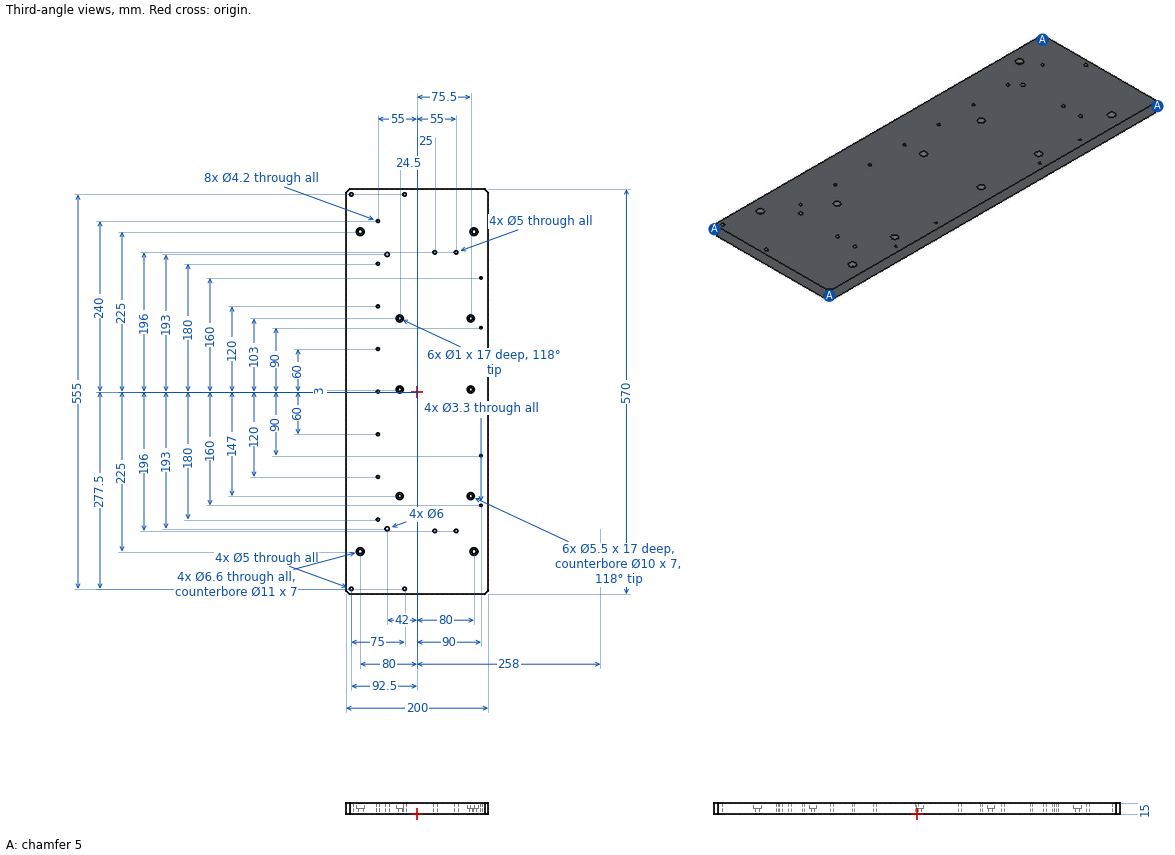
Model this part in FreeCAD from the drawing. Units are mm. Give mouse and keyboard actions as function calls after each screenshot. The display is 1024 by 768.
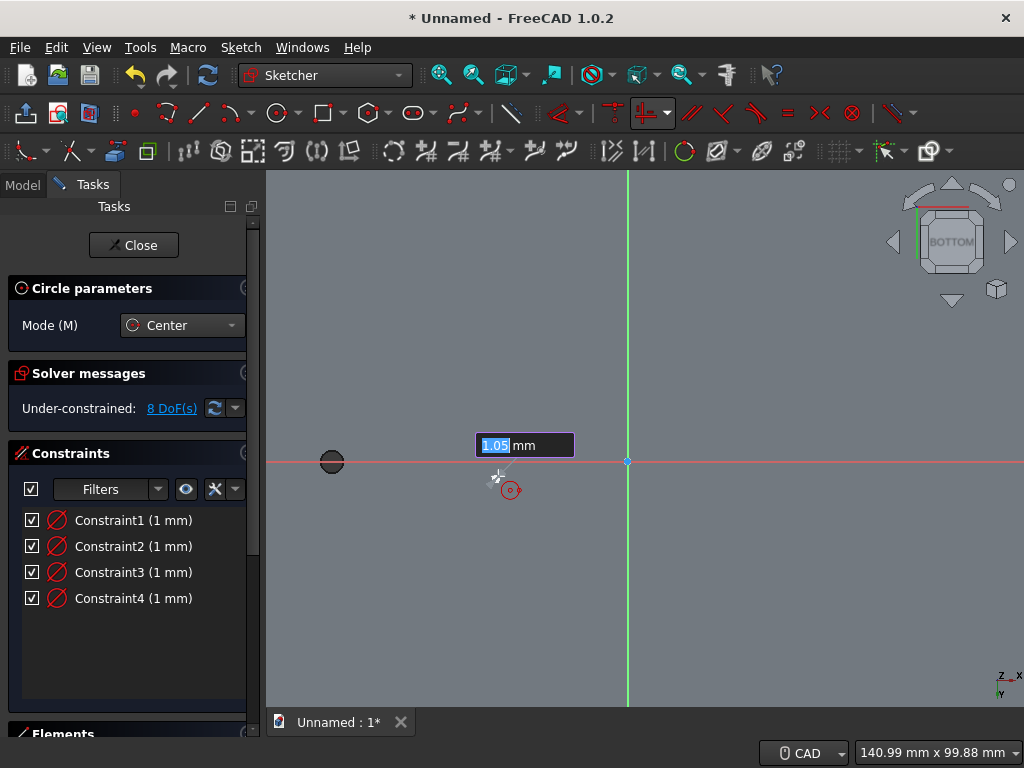
text(1)
key(Return)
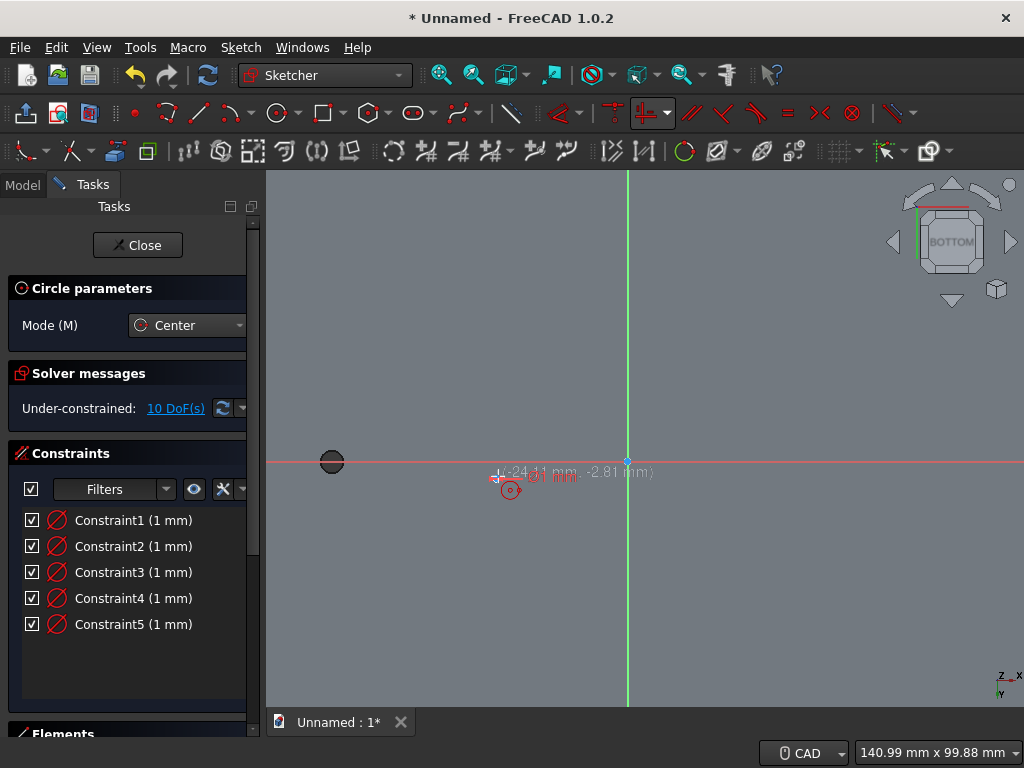
scroll(515, 470, down, 7)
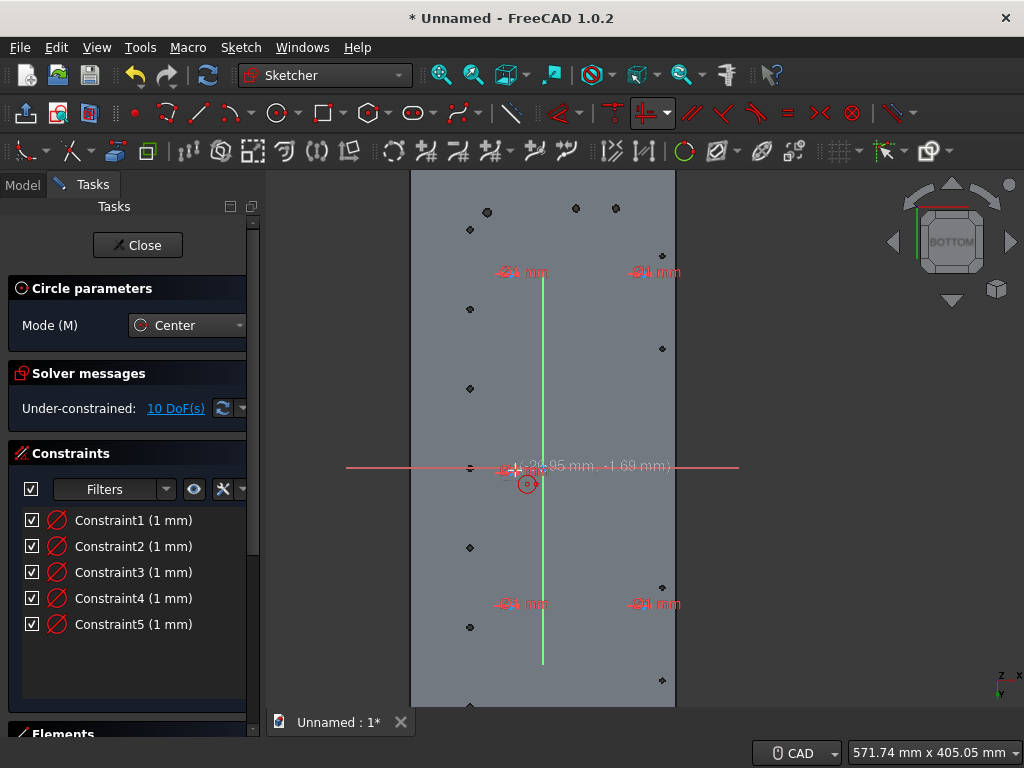
scroll(643, 472, up, 18)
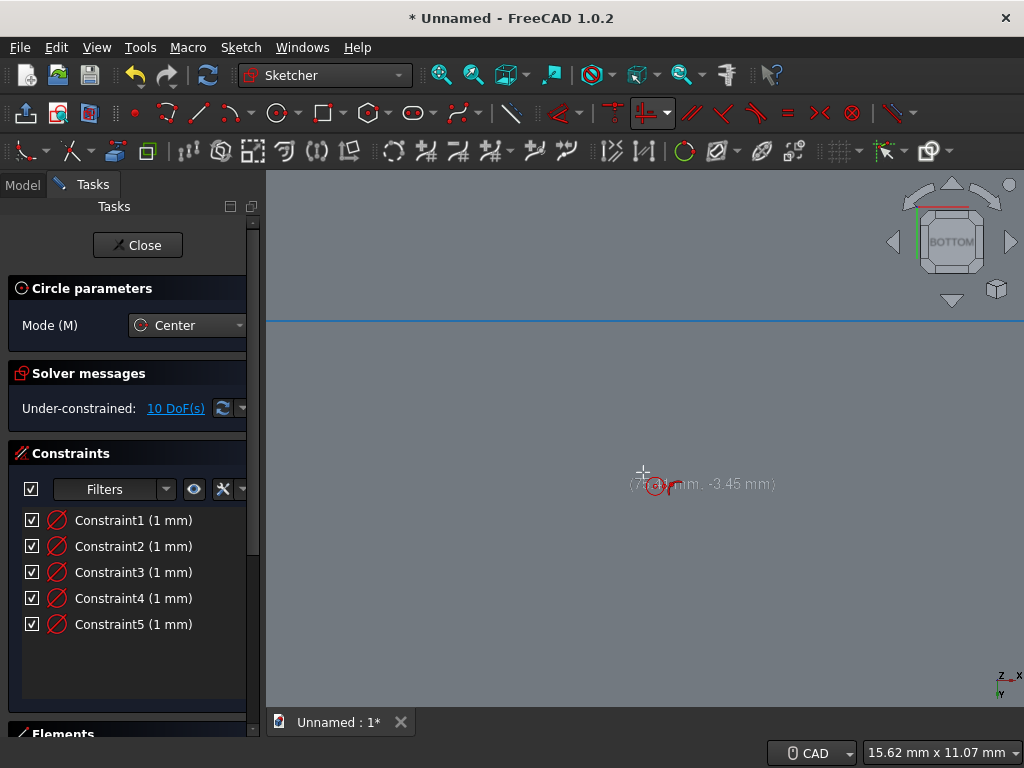
scroll(658, 479, down, 17)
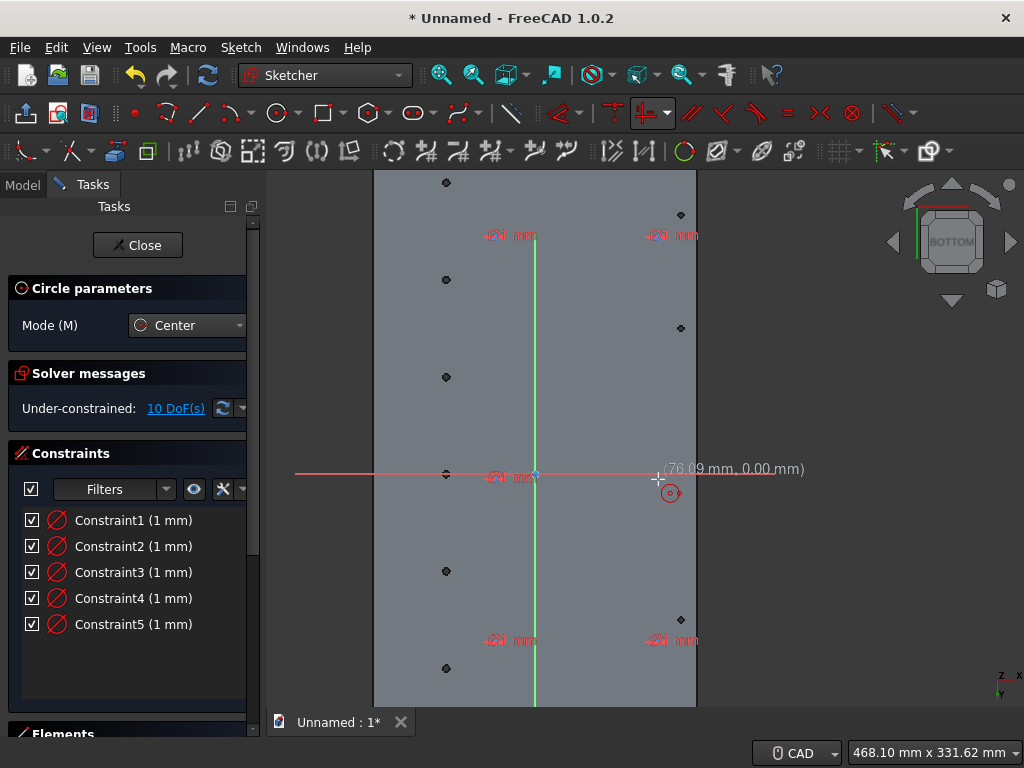
scroll(658, 479, up, 6)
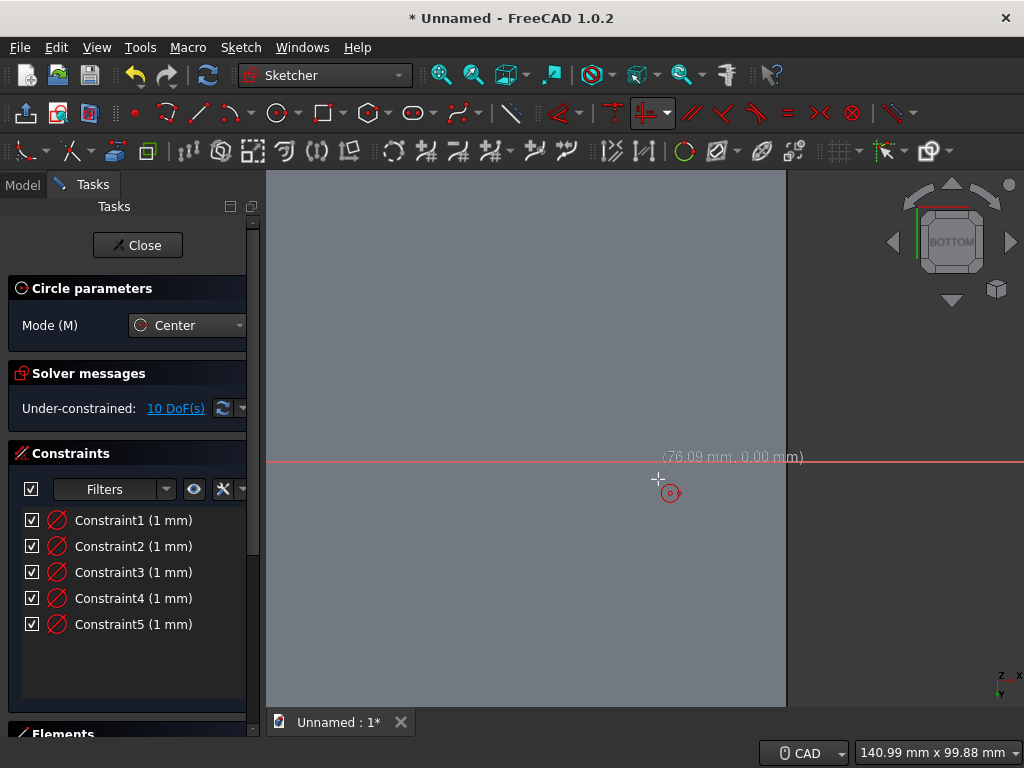
click(655, 478)
move(657, 476)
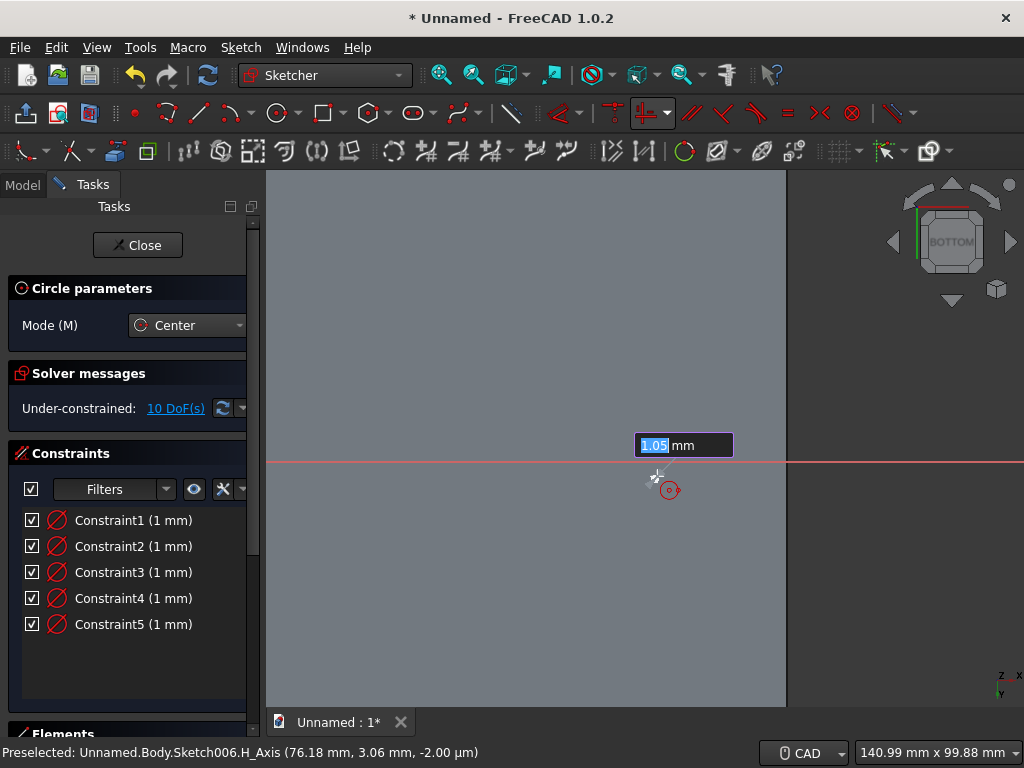
text(1)
key(Return)
key(Escape)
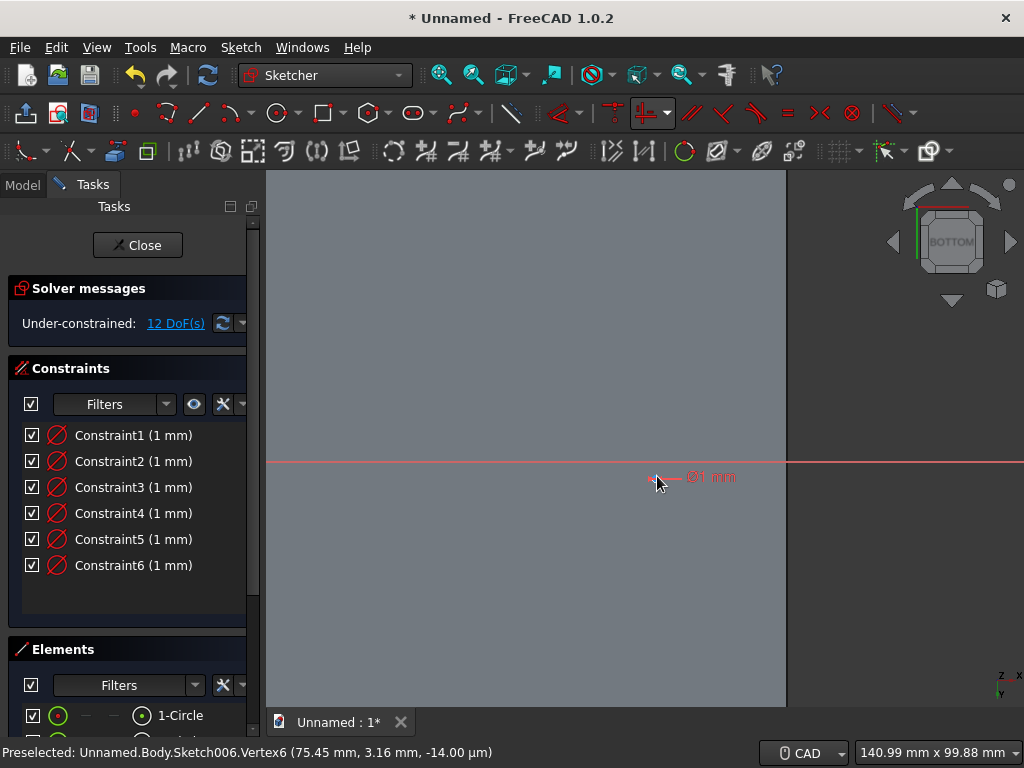
scroll(639, 470, down, 7)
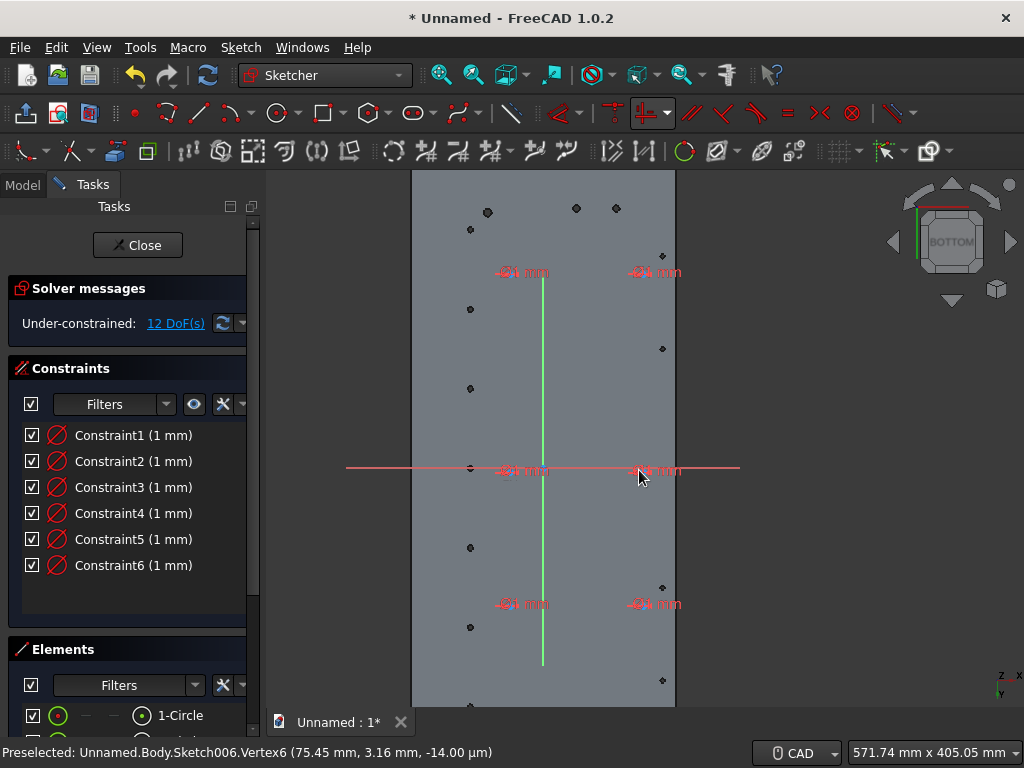
click(511, 606)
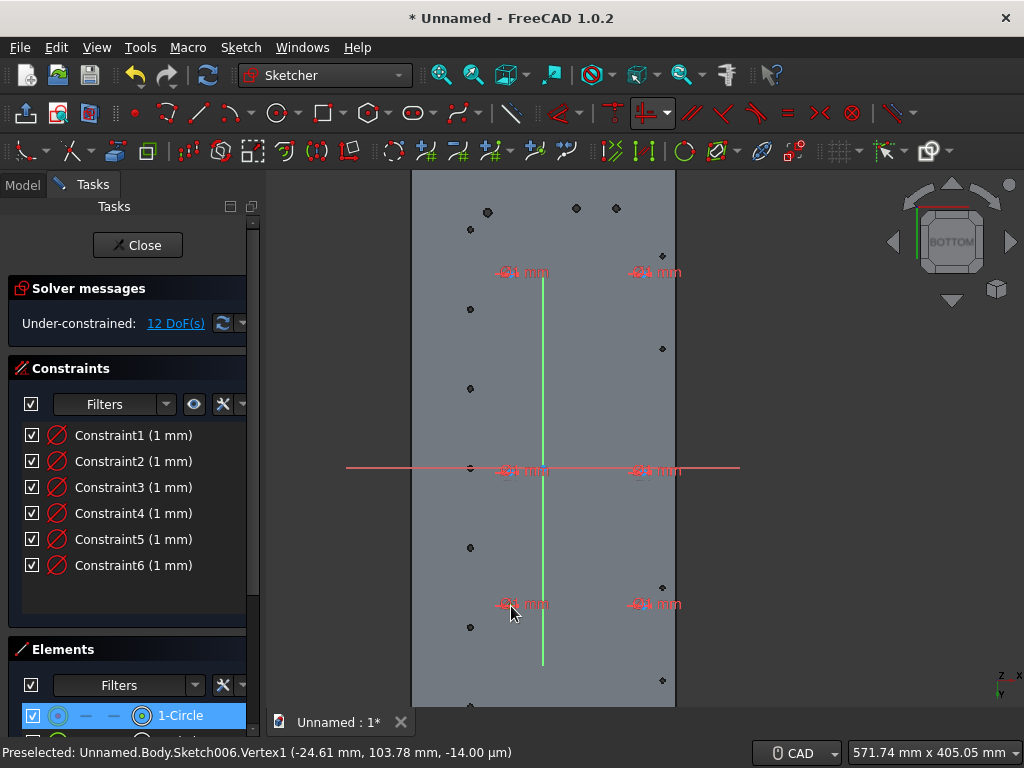
click(643, 606)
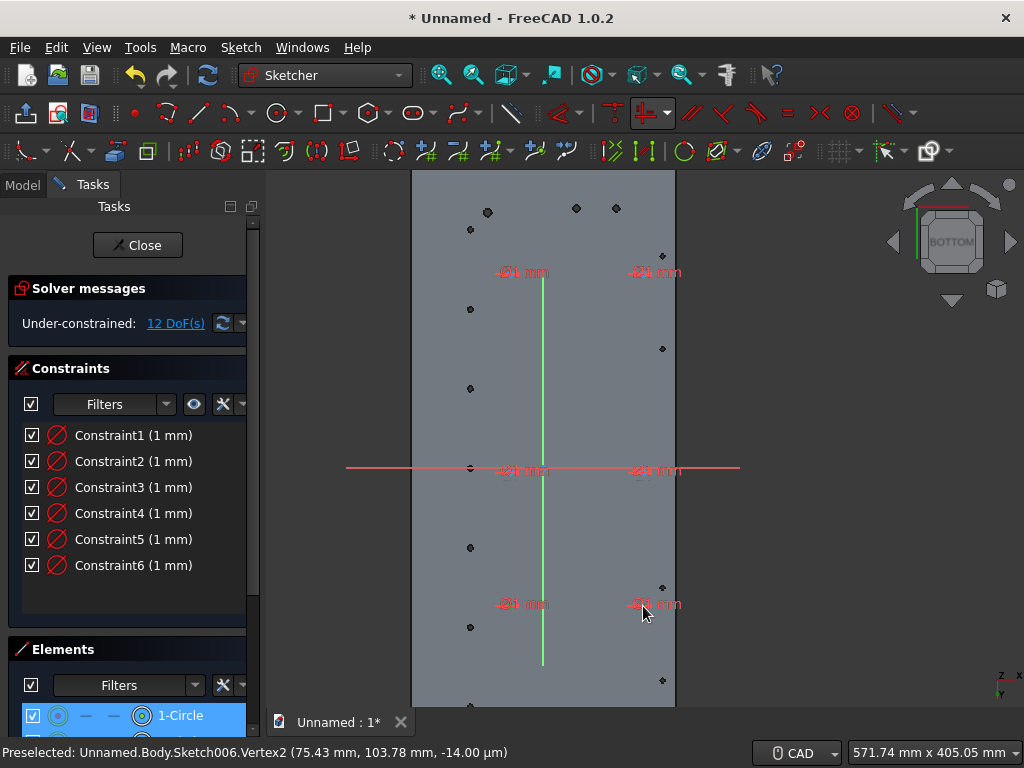
key(h)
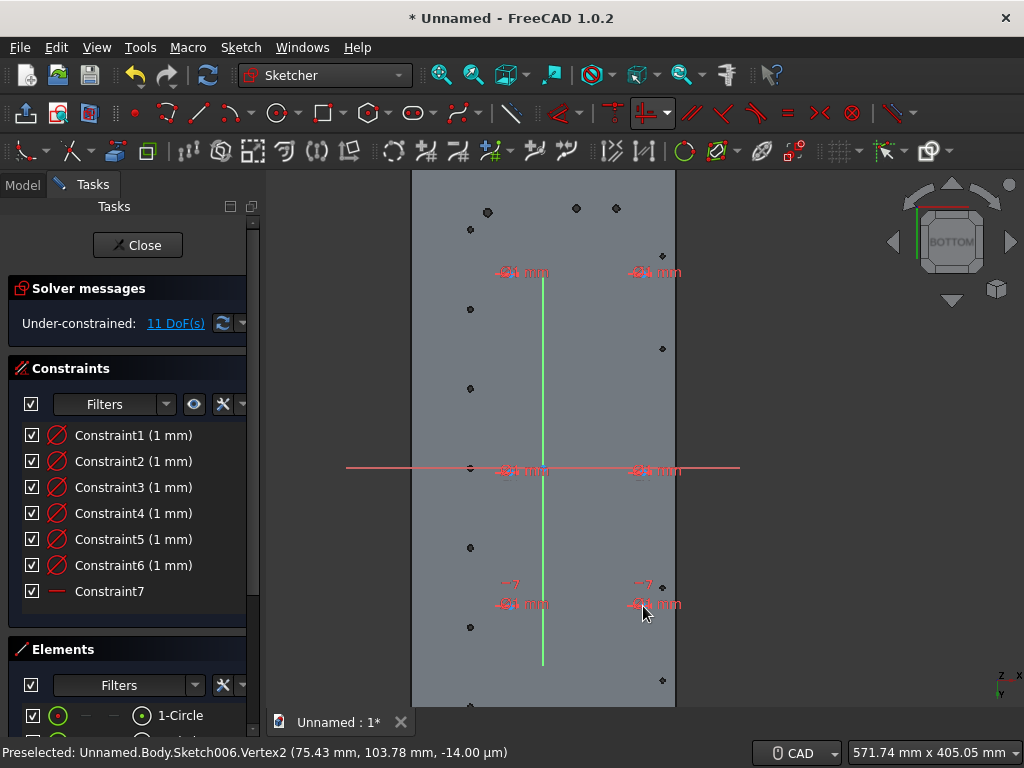
click(511, 606)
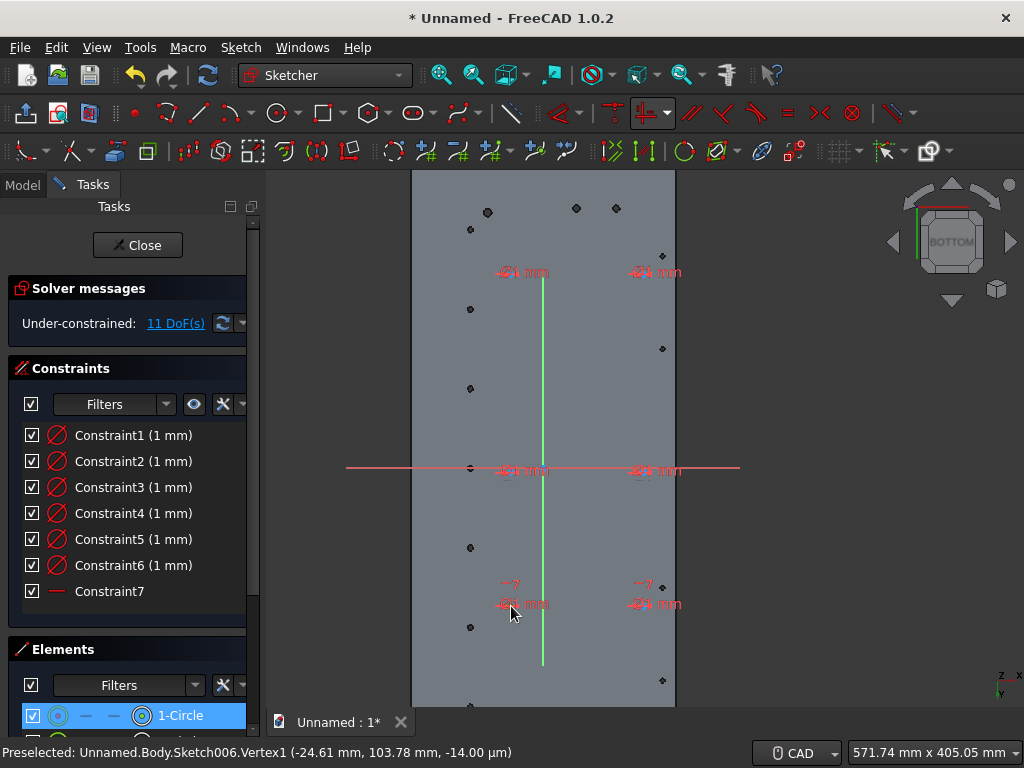
click(511, 274)